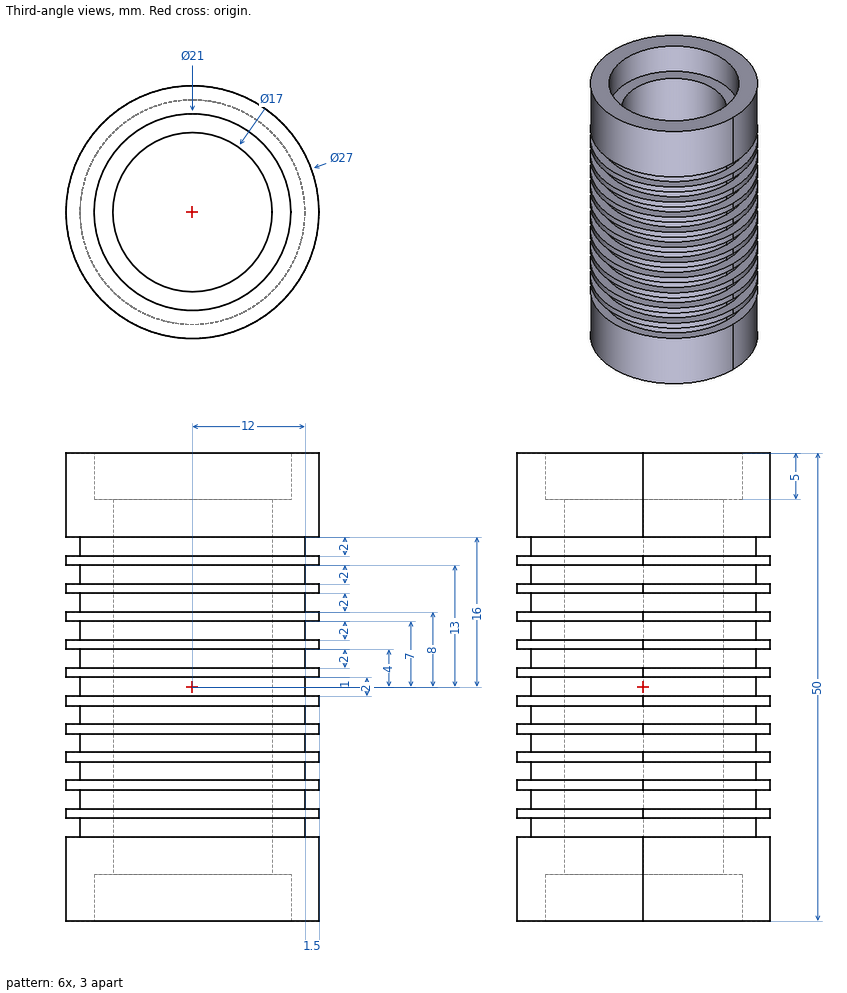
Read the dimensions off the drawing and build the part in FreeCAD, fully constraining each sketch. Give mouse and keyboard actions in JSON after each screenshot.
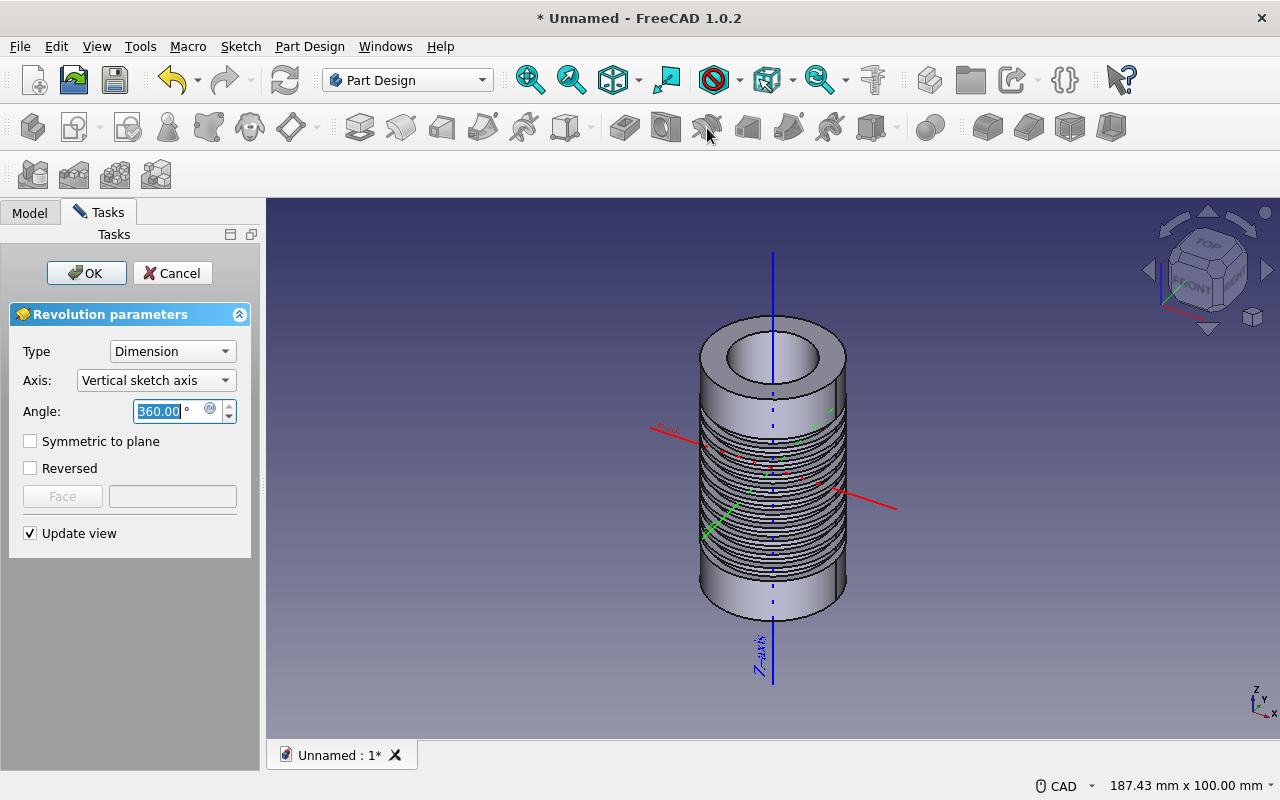
{"action": "left_click", "coordinate": [87, 273]}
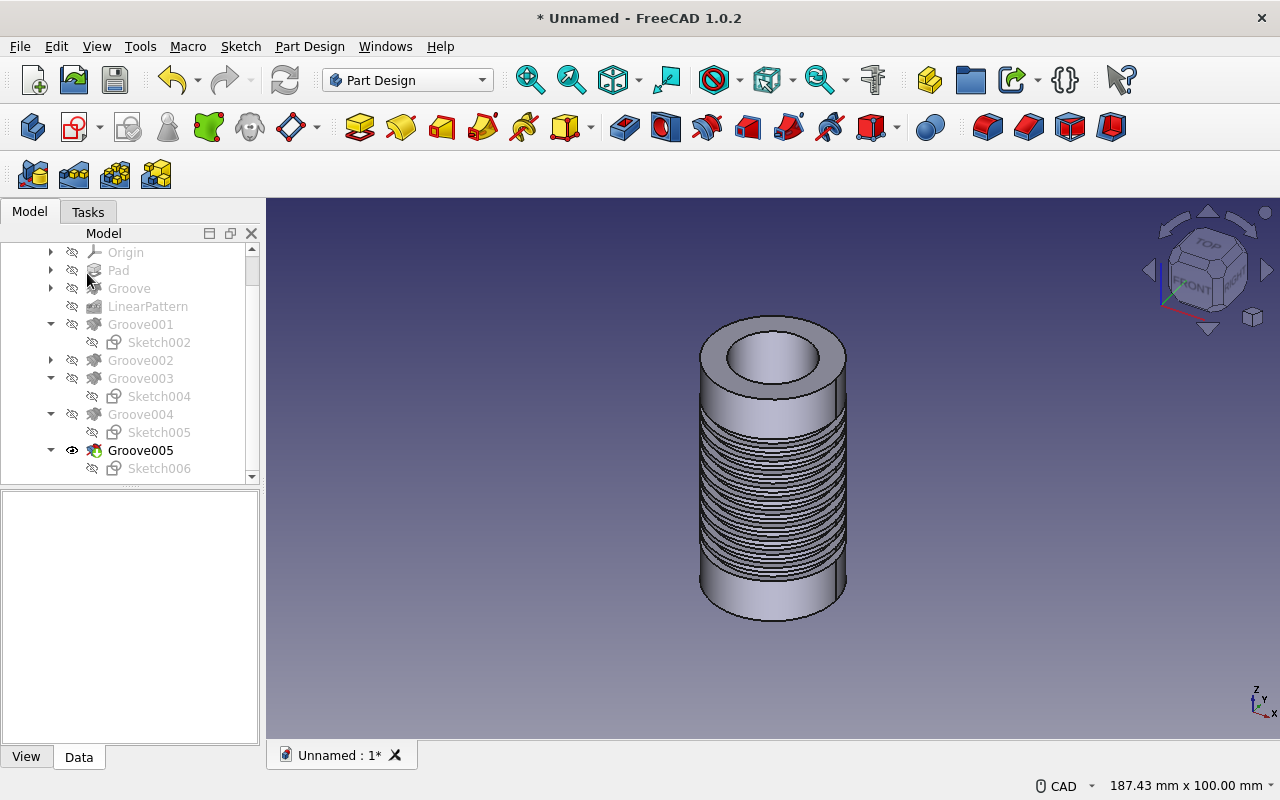
{"action": "left_click", "coordinate": [830, 348]}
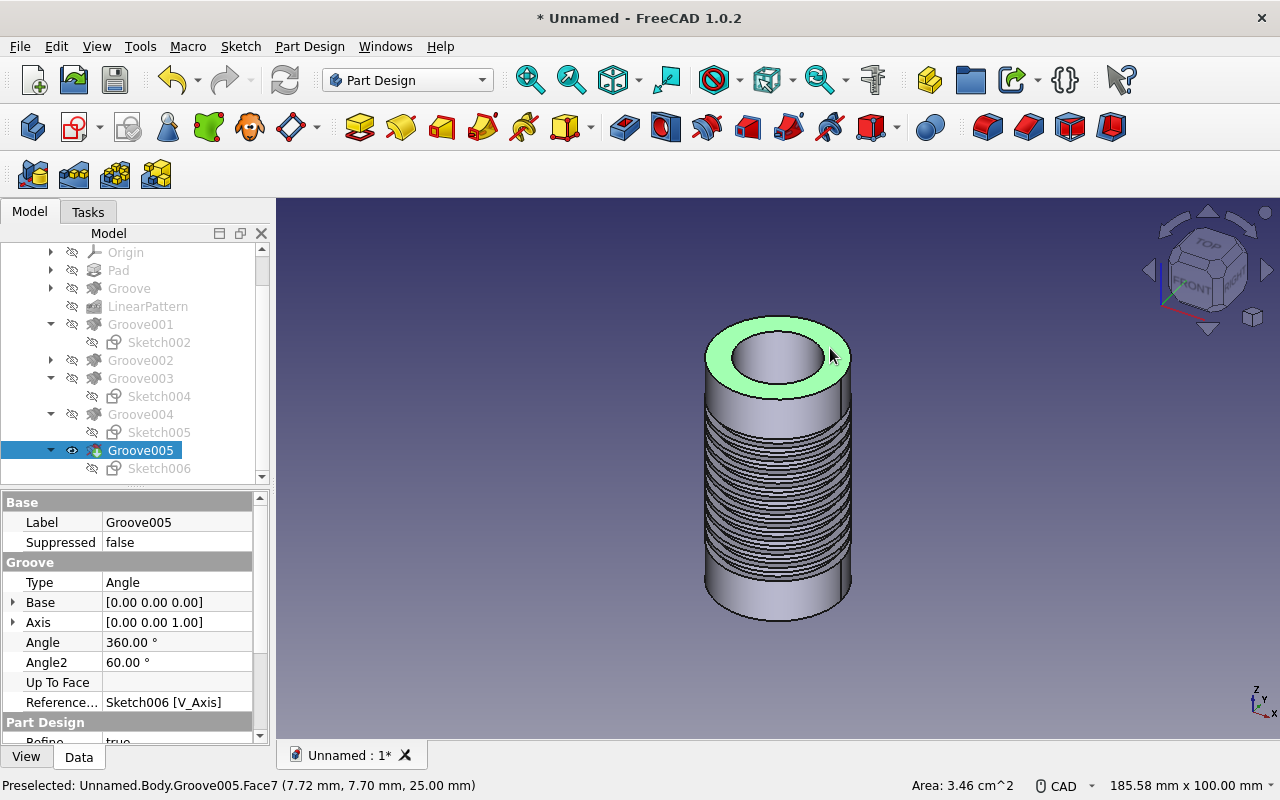
{"action": "left_click", "coordinate": [74, 128]}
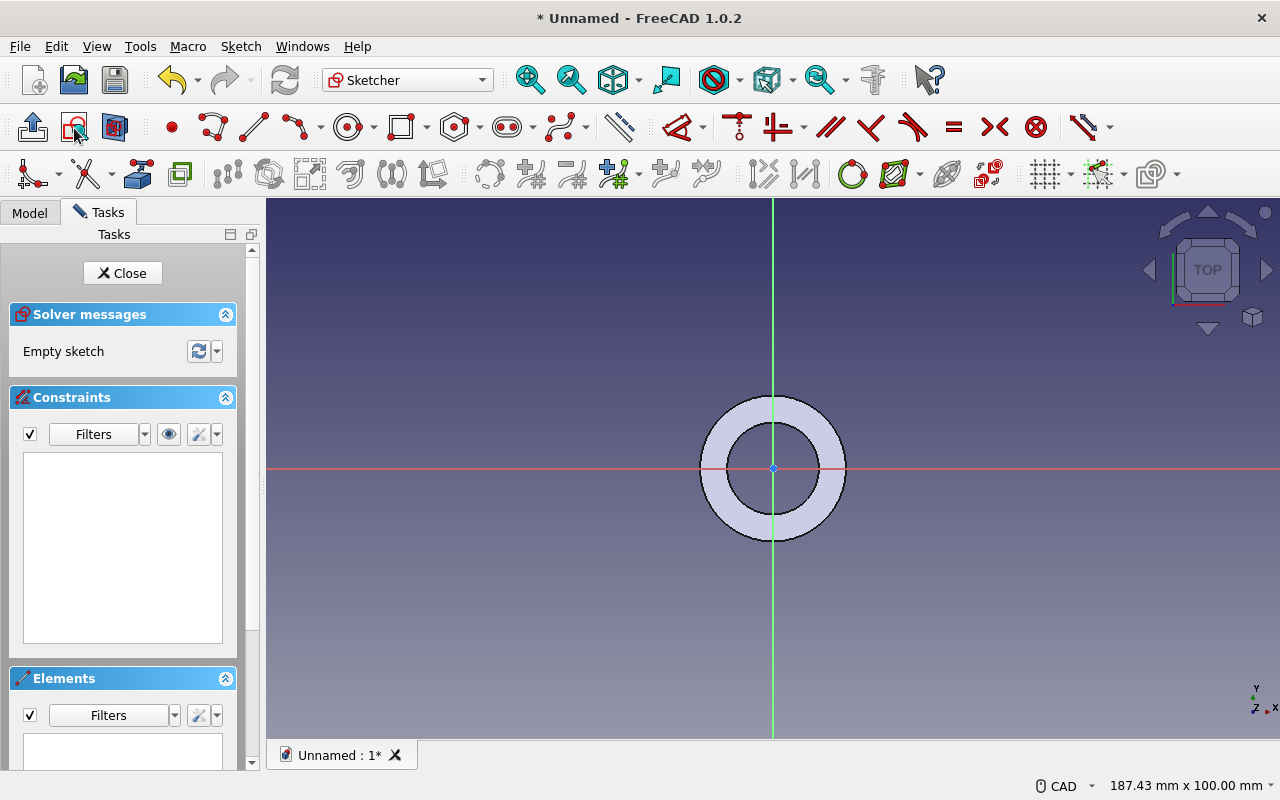
{"action": "scroll", "coordinate": [803, 468], "scroll_direction": "up", "scroll_amount": 6}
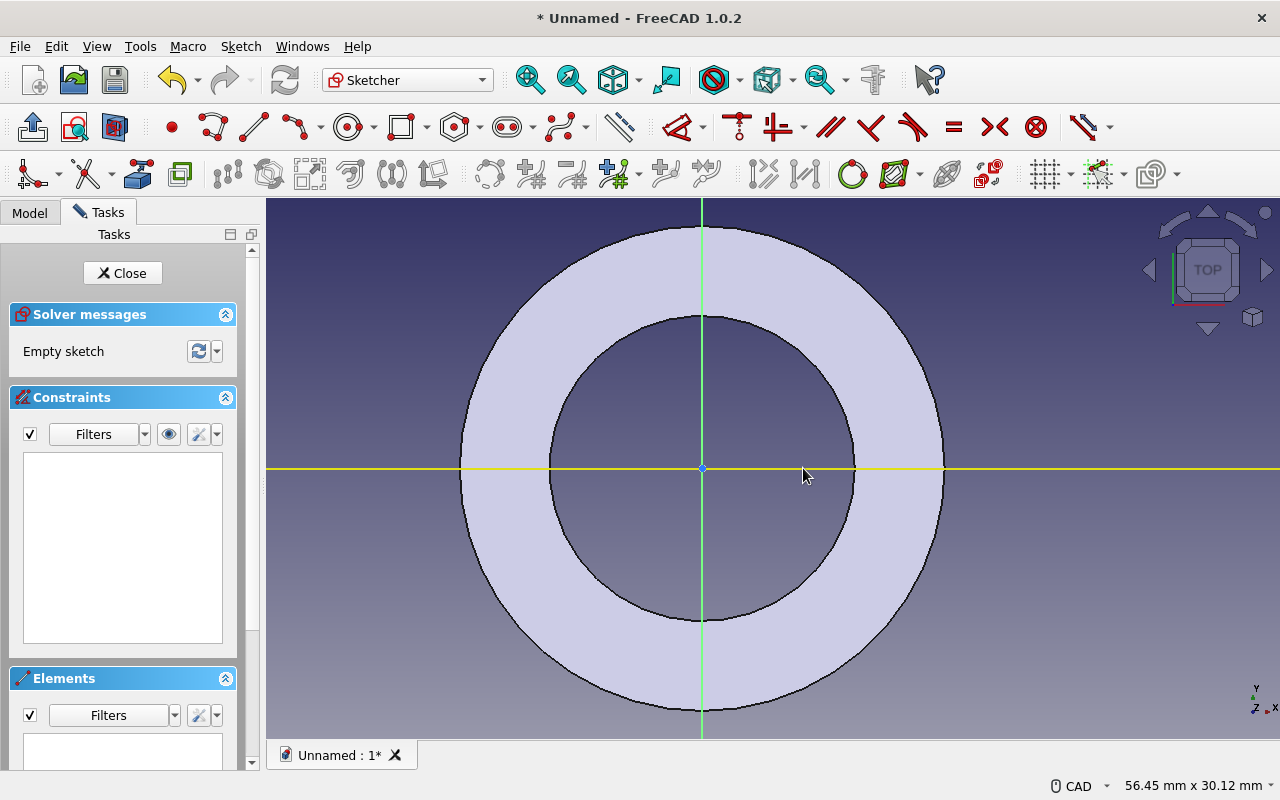
{"action": "left_click", "coordinate": [348, 128]}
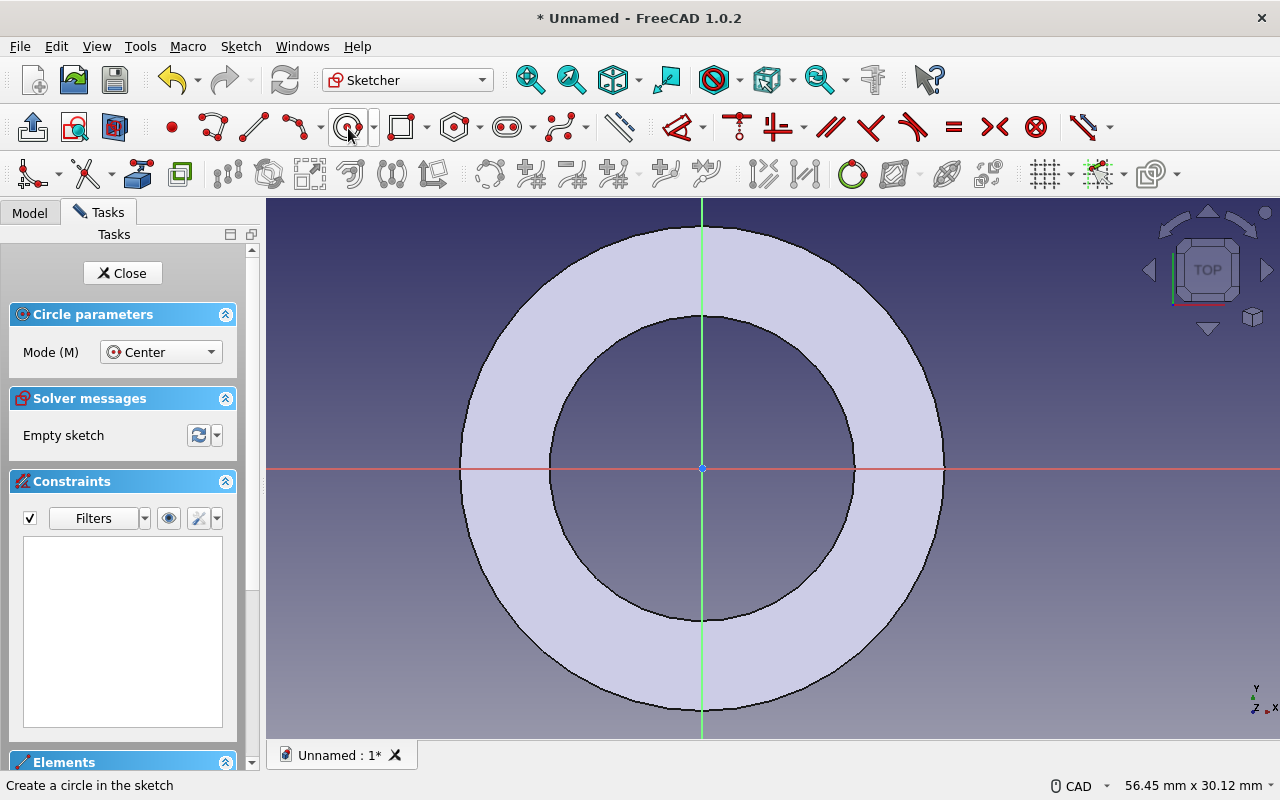
{"action": "left_click", "coordinate": [702, 468]}
{"action": "mouse_move", "coordinate": [836, 335]}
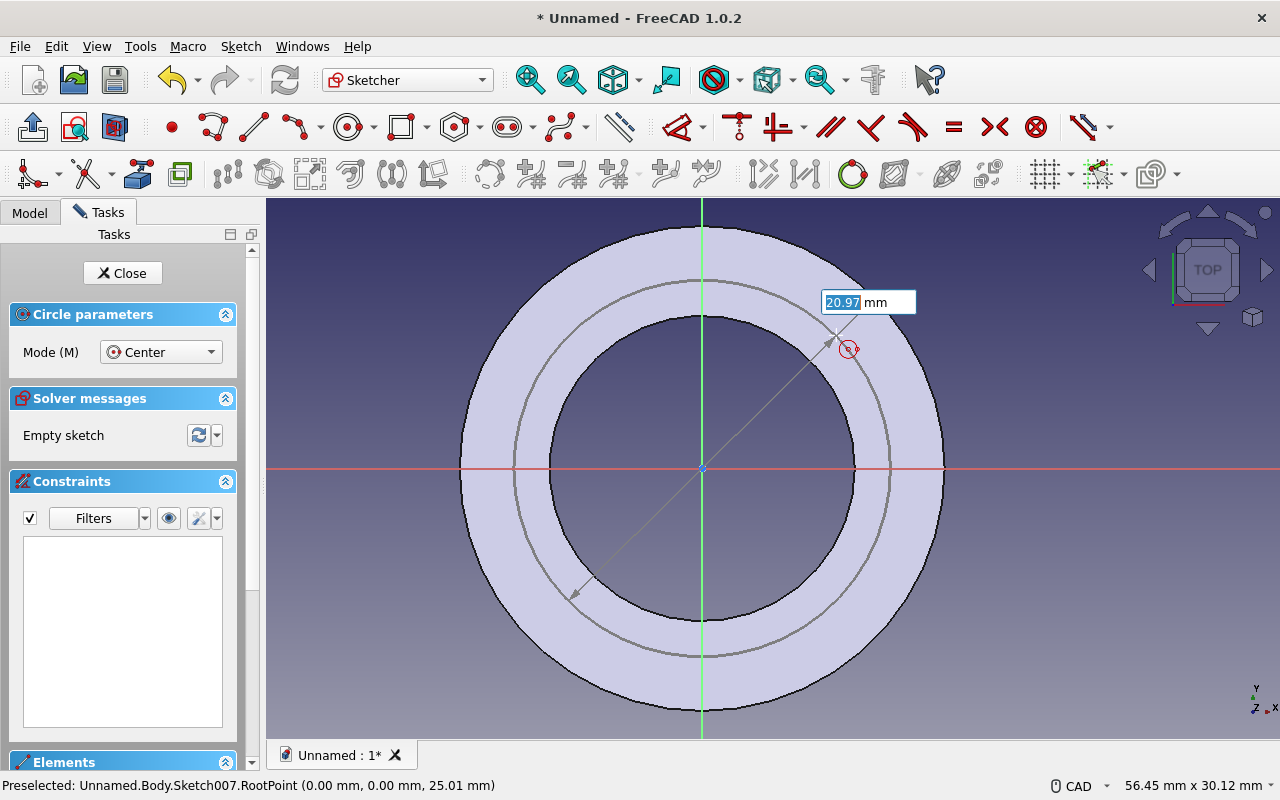
{"action": "type", "text": "21"}
{"action": "key", "text": "Return"}
{"action": "key", "text": "Escape"}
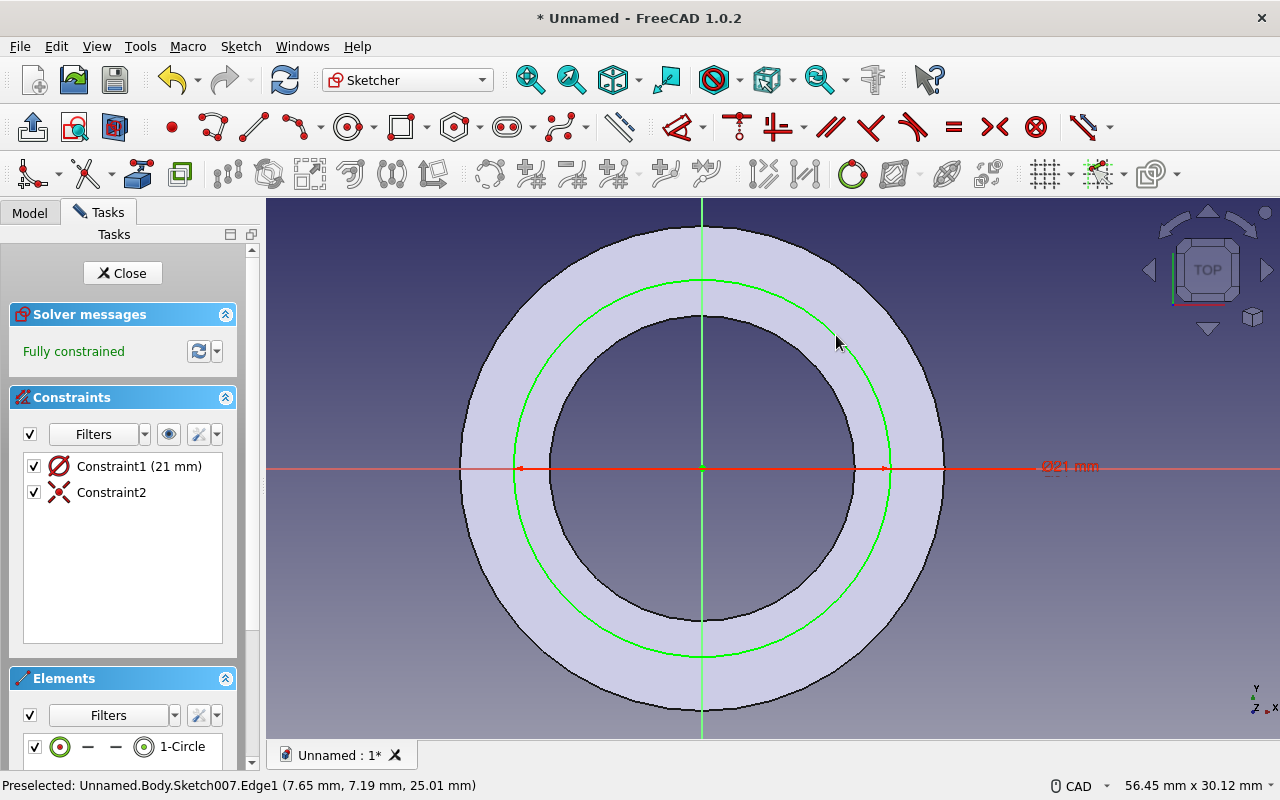
{"action": "left_click", "coordinate": [123, 273]}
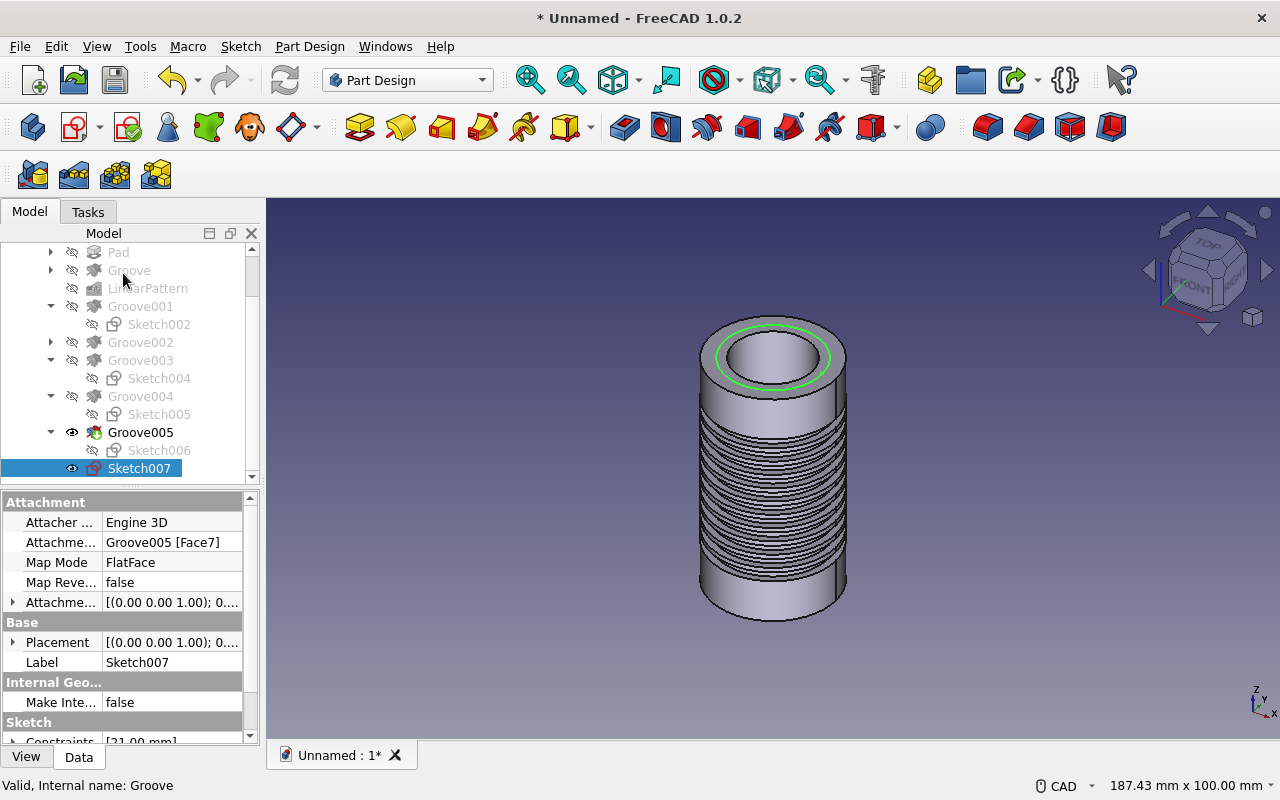
{"action": "left_click", "coordinate": [625, 128]}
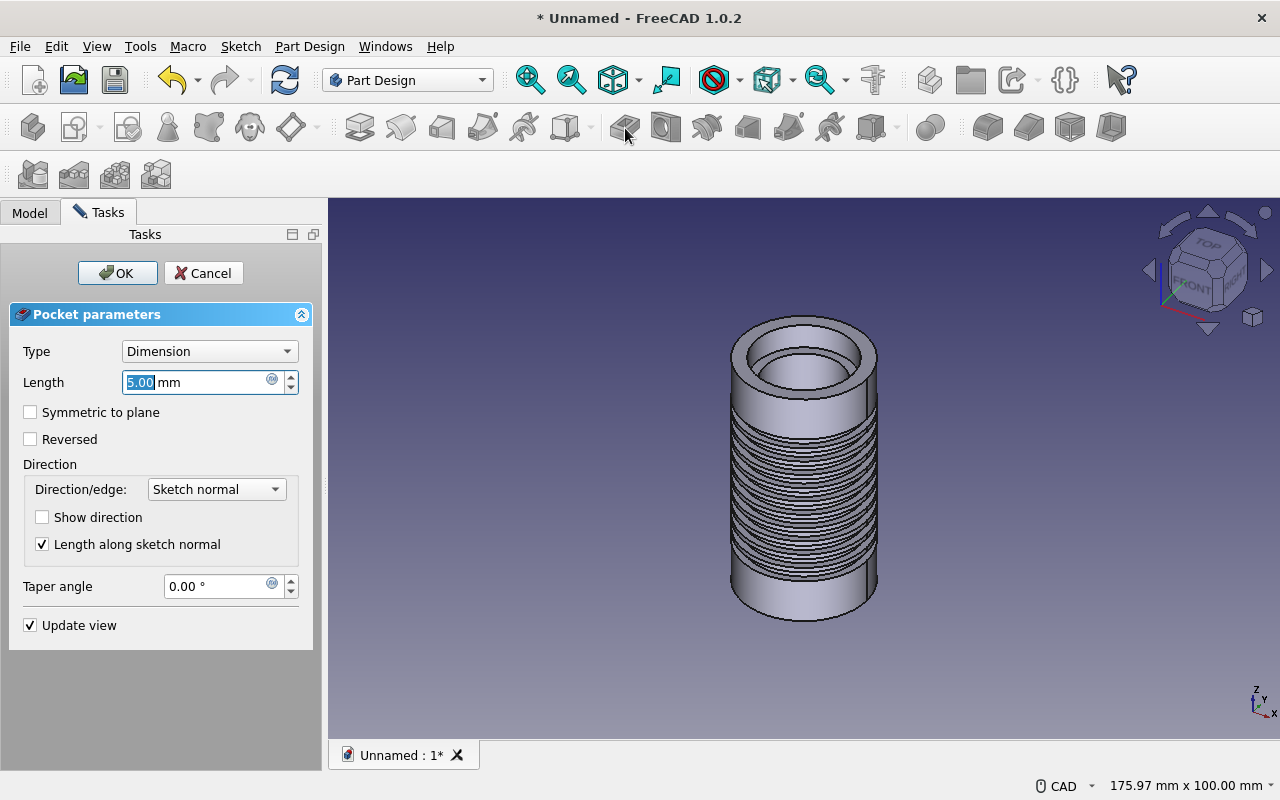
{"action": "type", "text": "5"}
{"action": "key", "text": "Tab"}